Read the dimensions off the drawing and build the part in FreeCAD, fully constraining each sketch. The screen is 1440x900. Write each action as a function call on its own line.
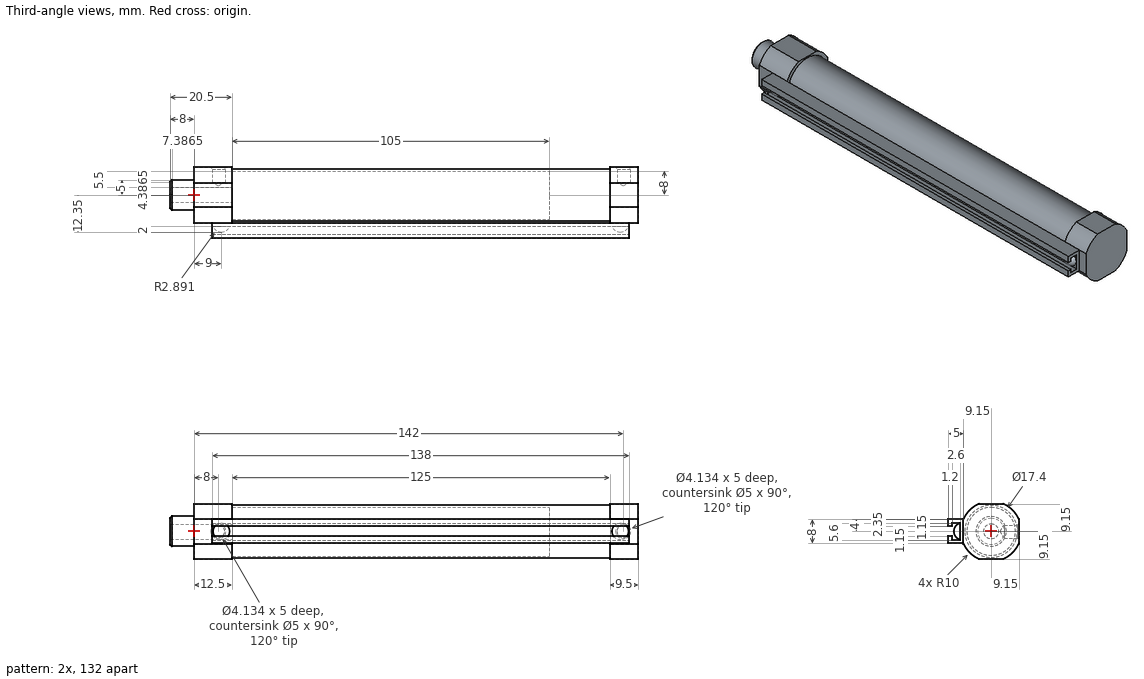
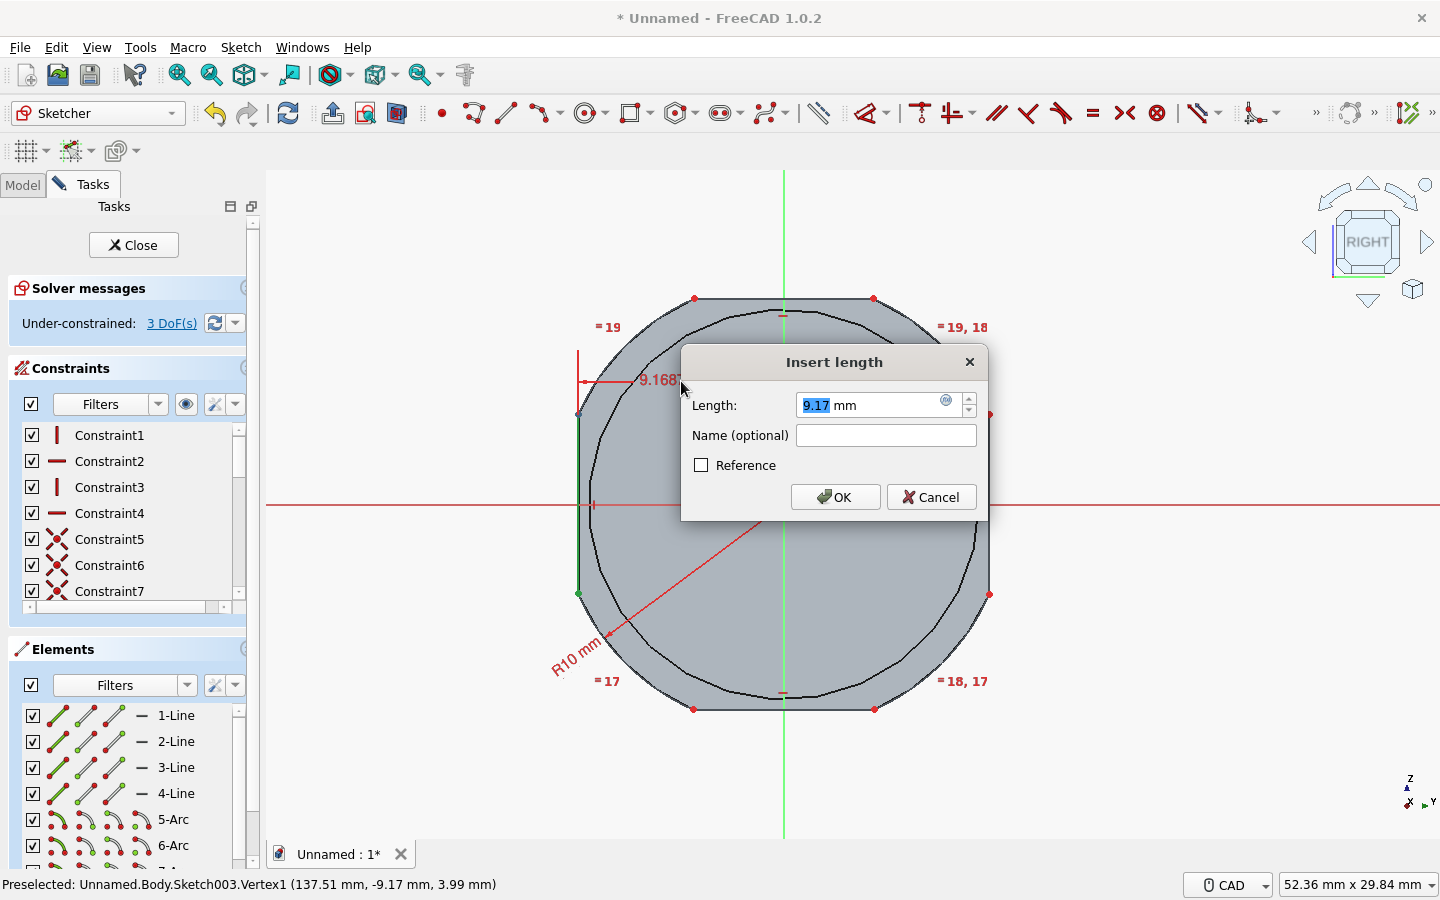
text(9.15)
key(Return)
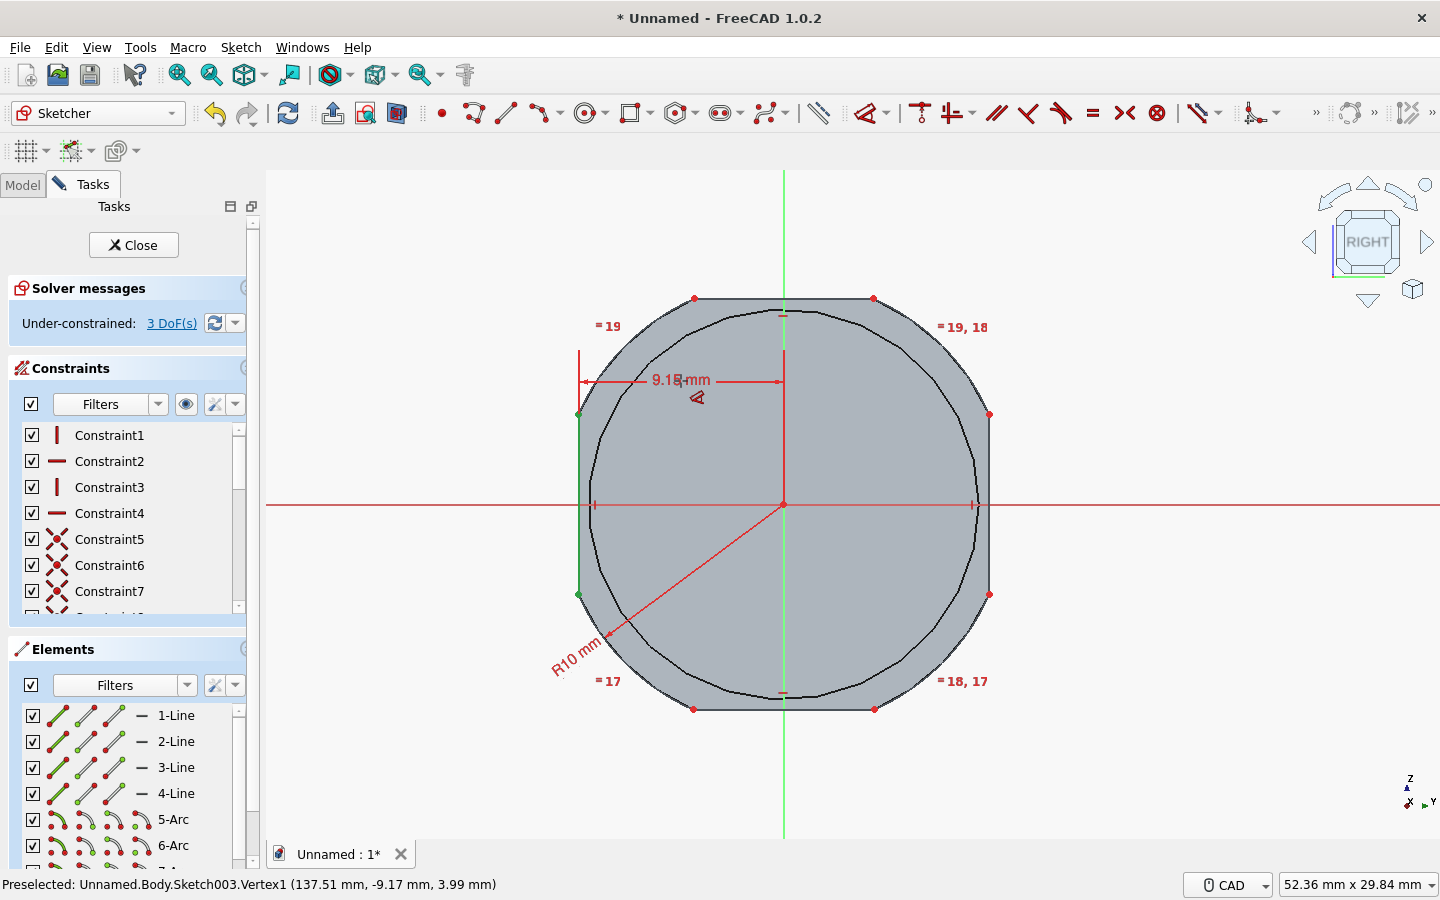
click(693, 710)
click(659, 607)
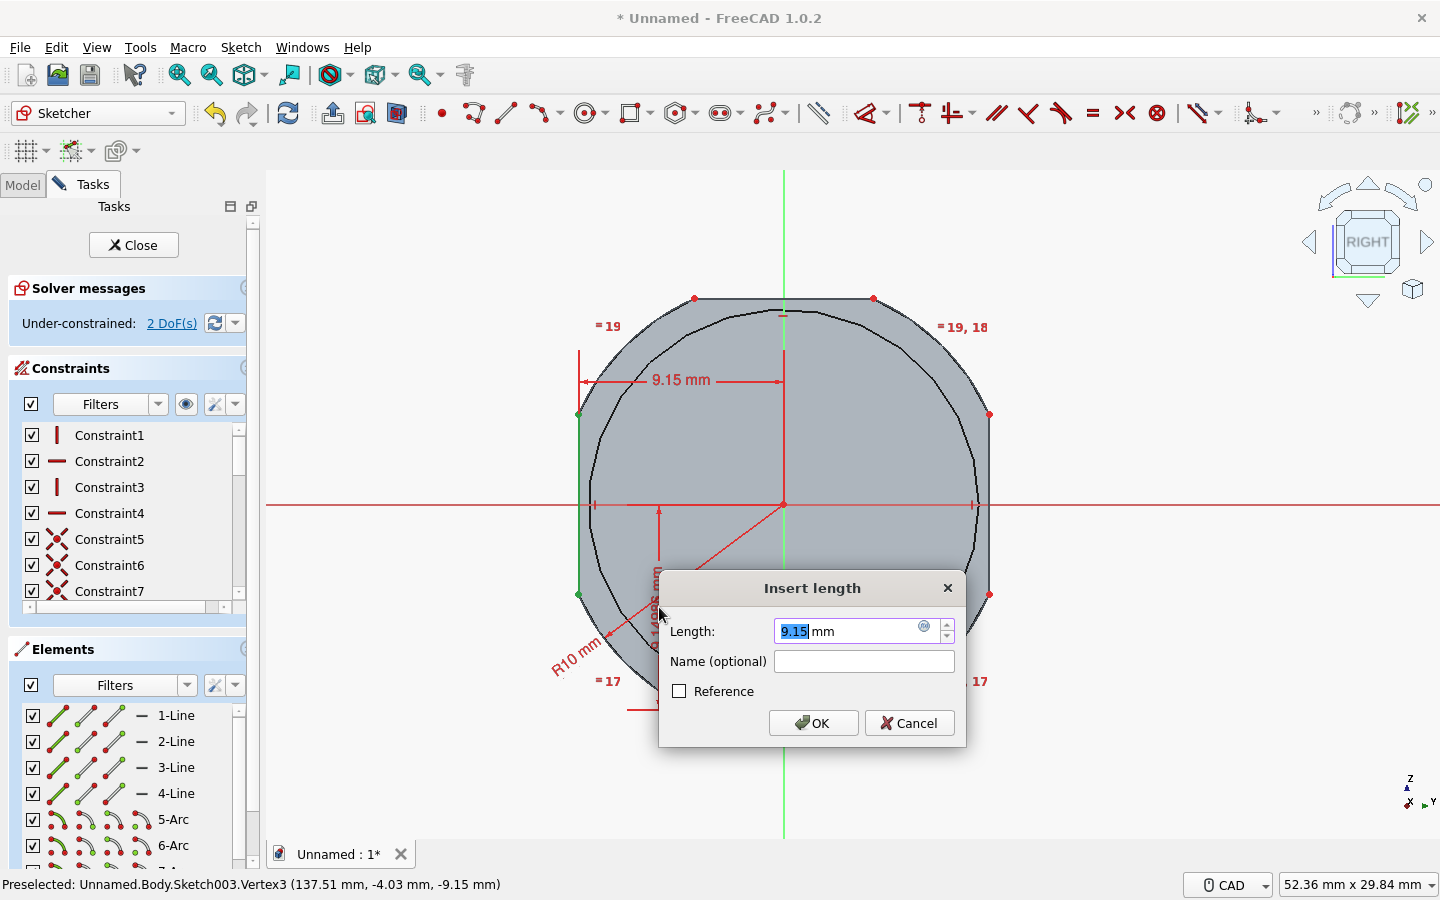
text(9.15)
key(Return)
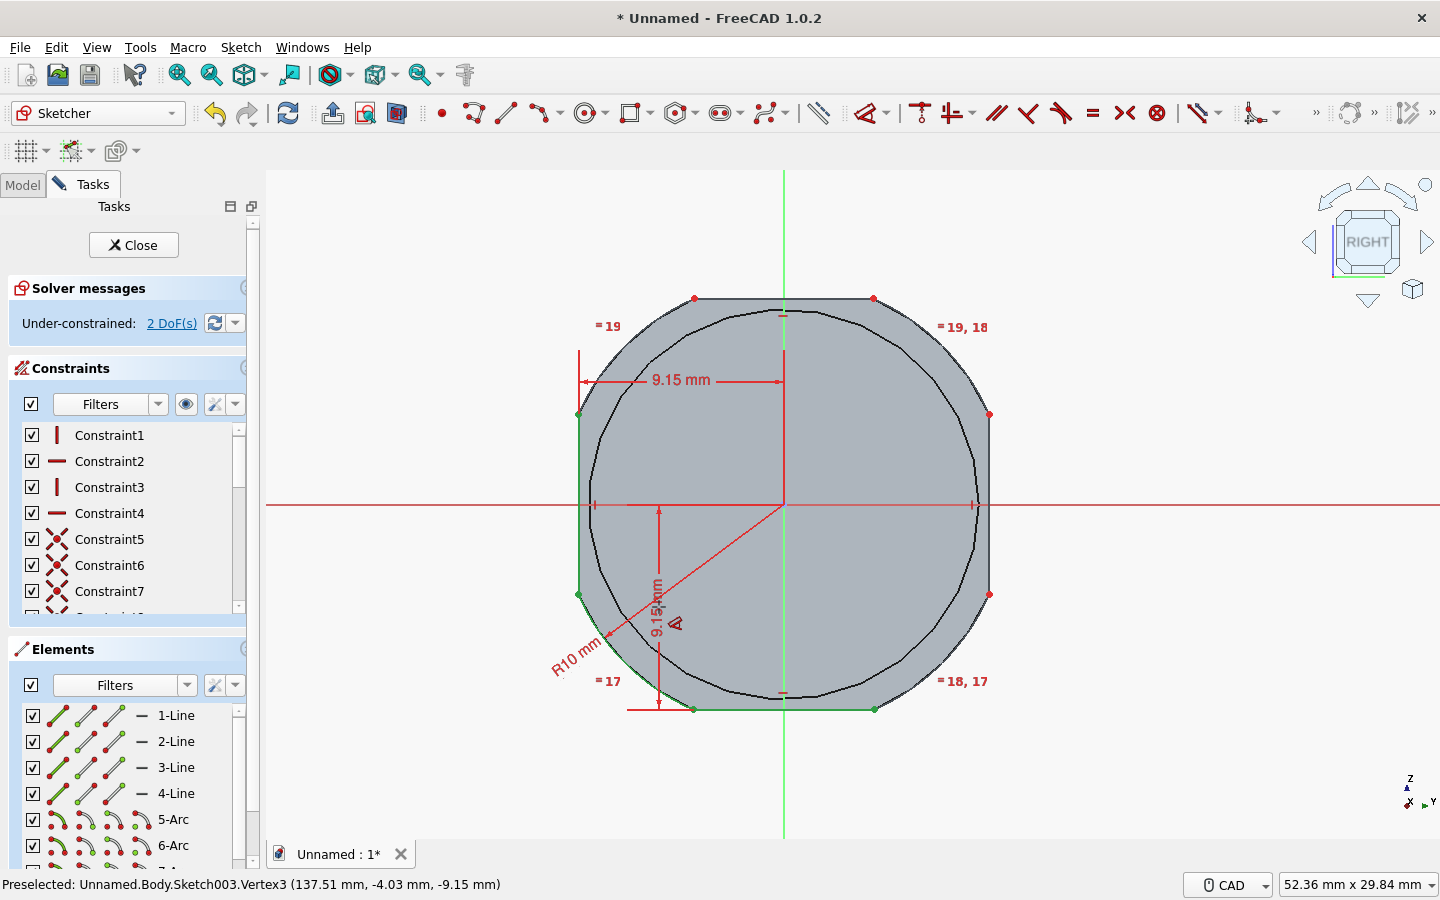
click(989, 594)
click(887, 628)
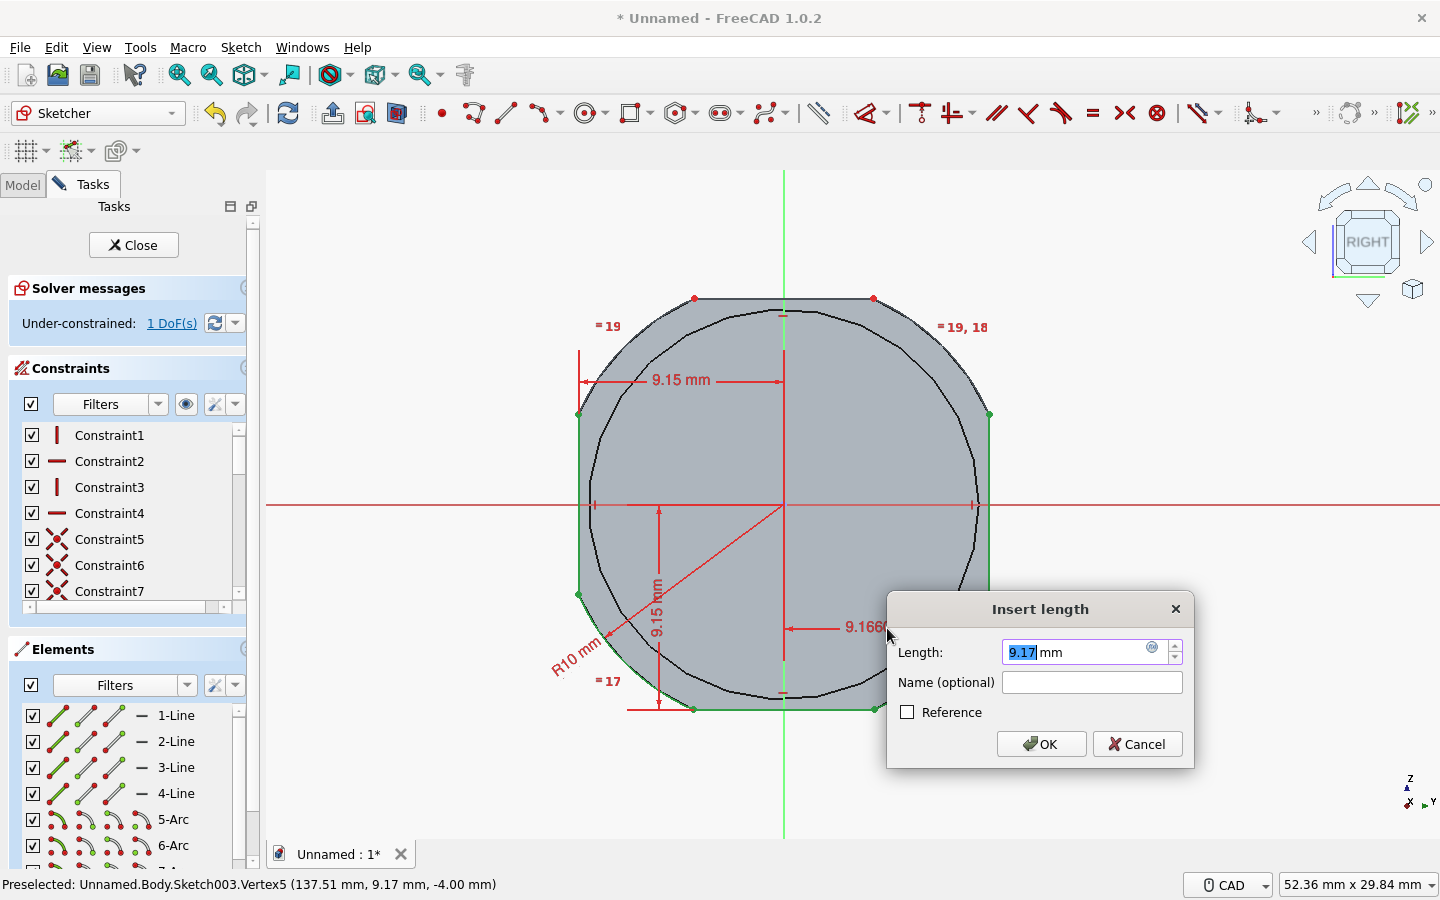
text(9.15)
key(Return)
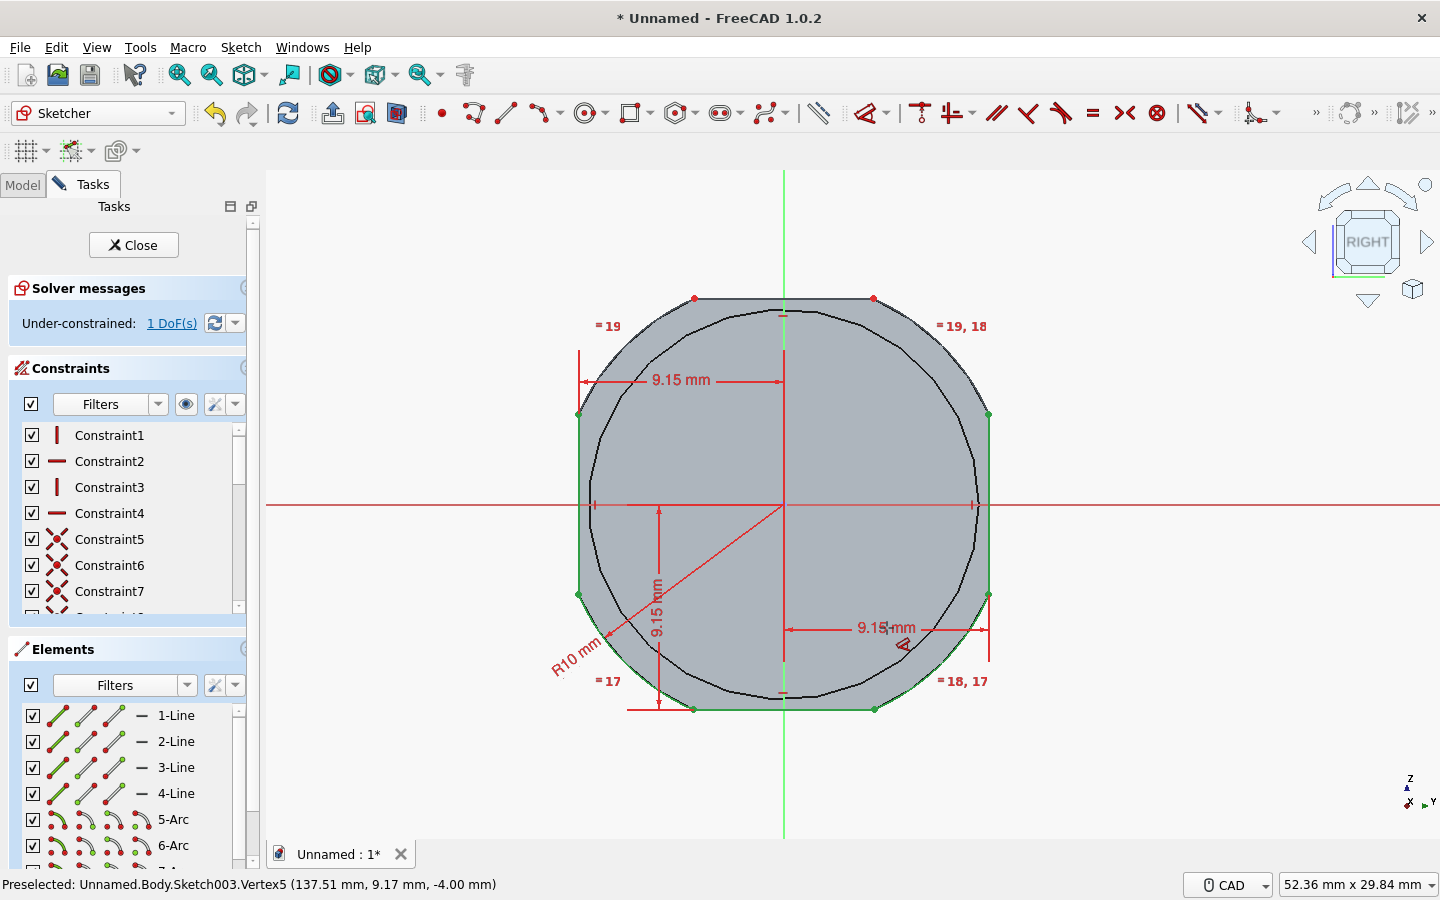
click(873, 299)
click(907, 402)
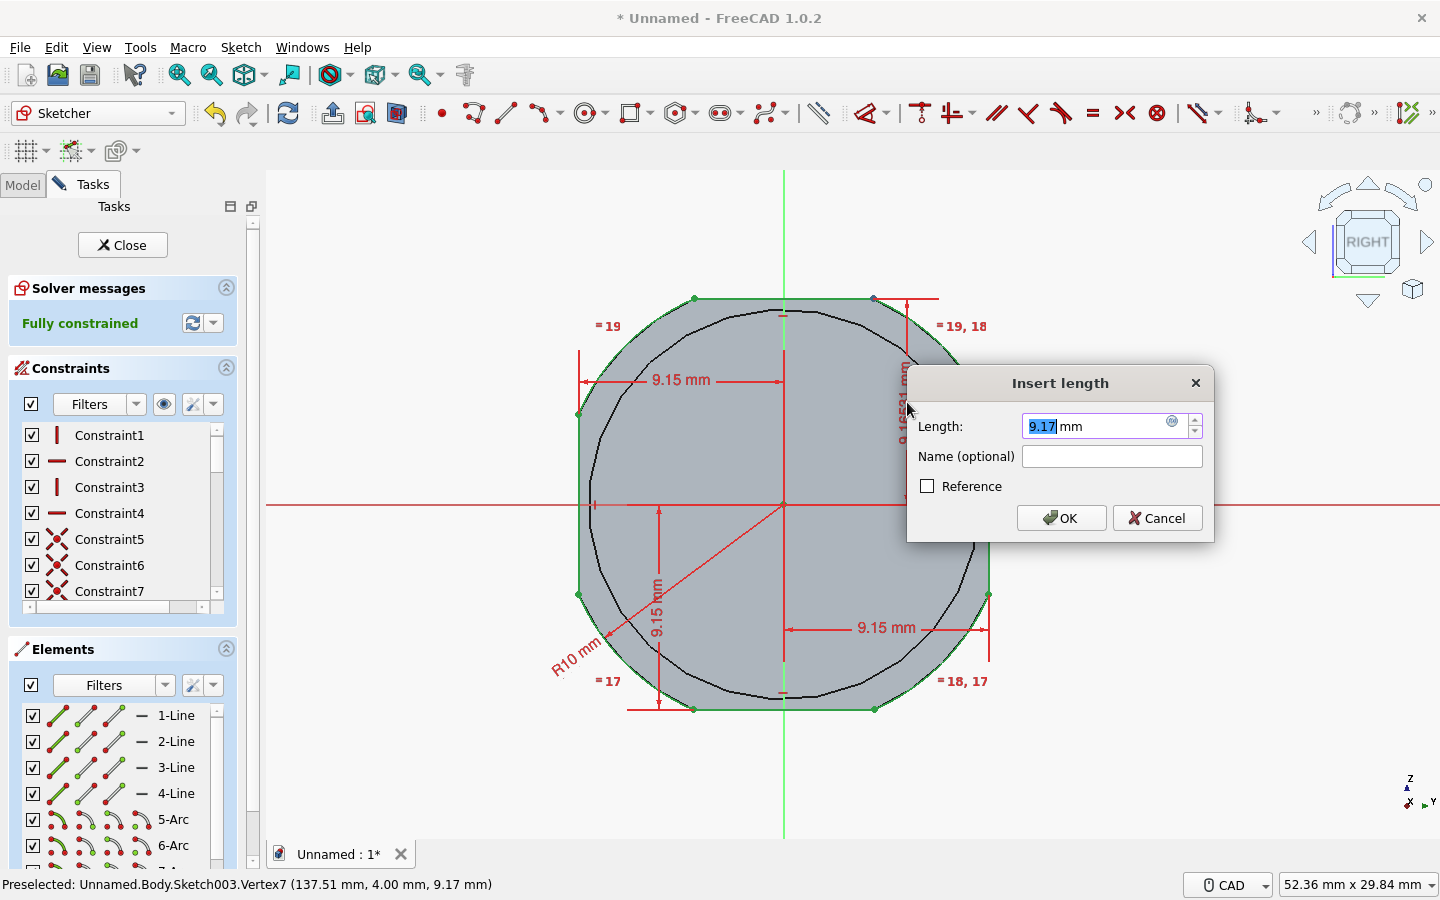
text(9.15)
key(Return)
key(Escape)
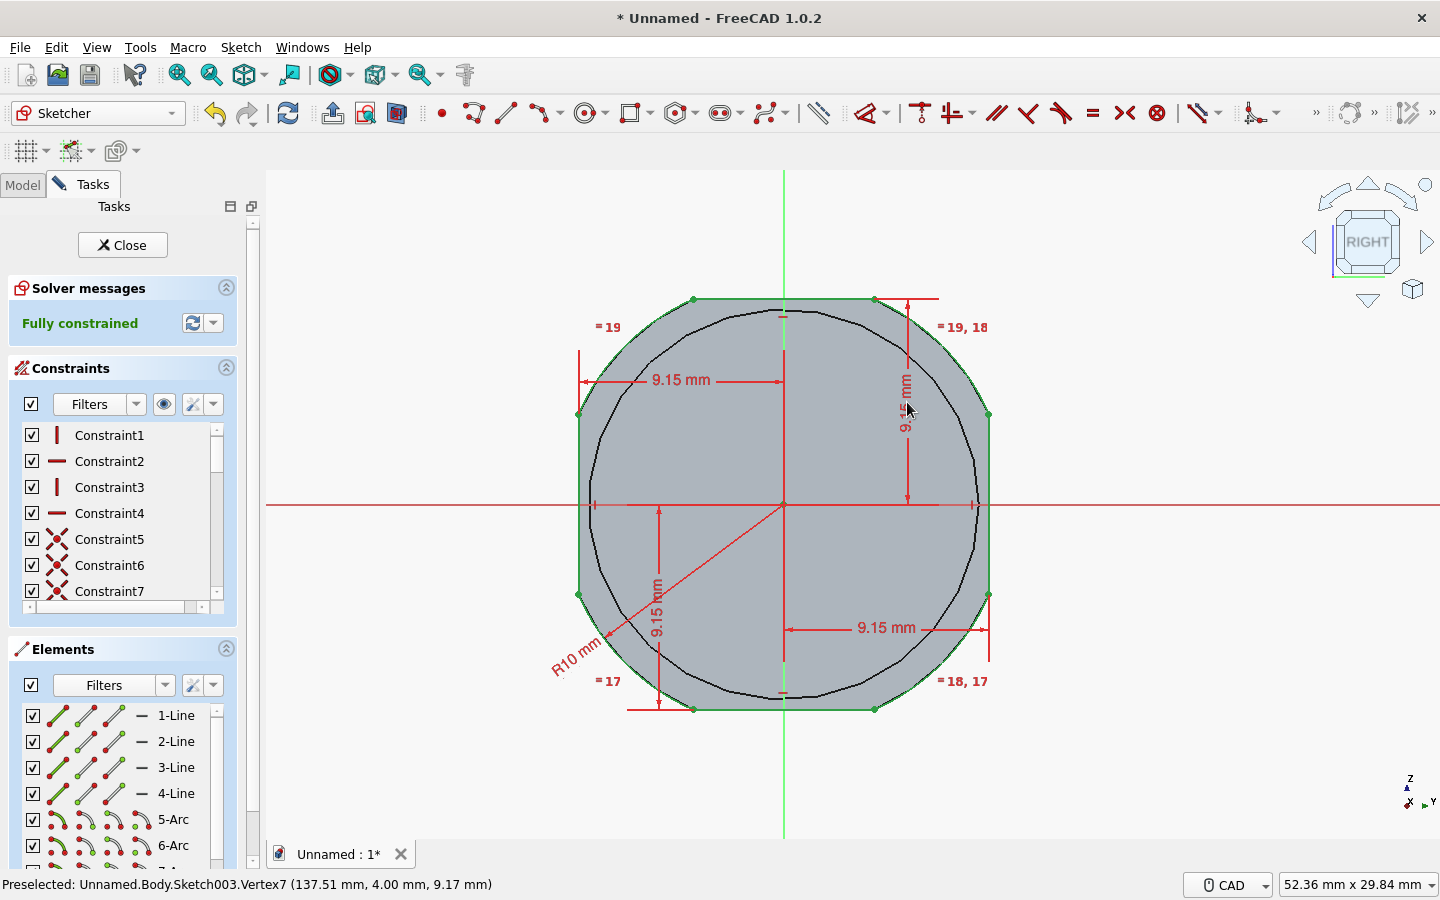
click(123, 245)